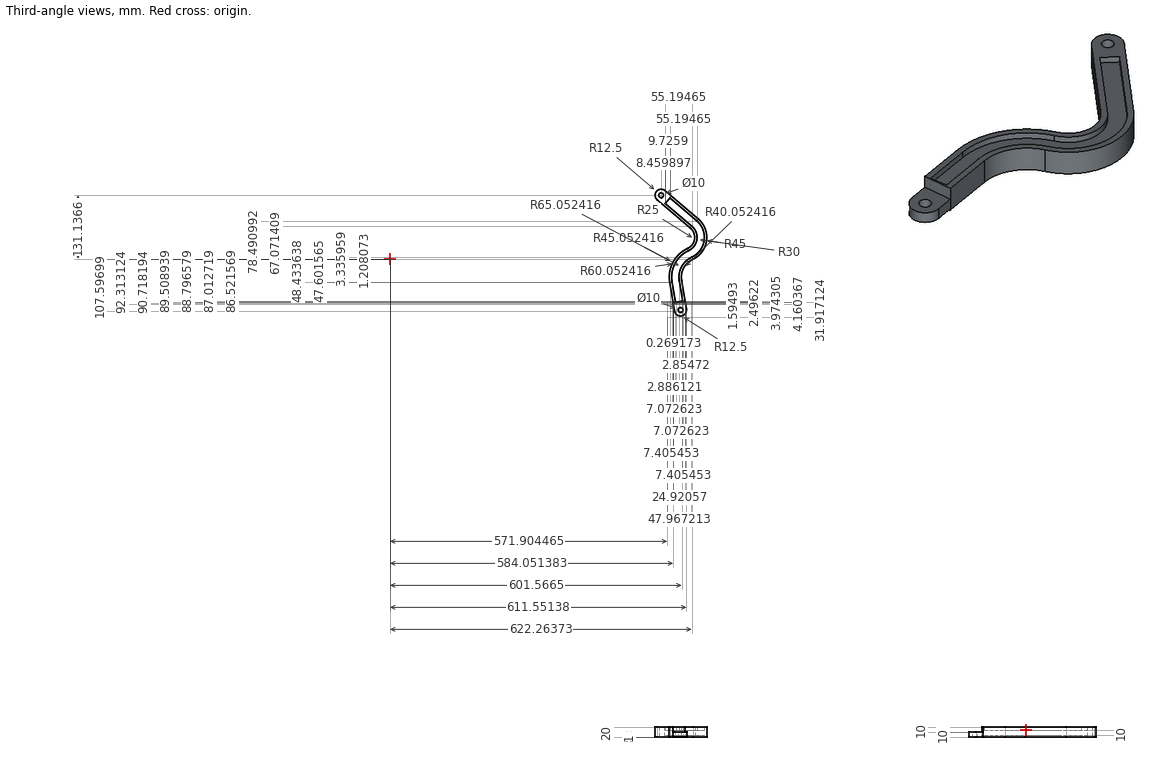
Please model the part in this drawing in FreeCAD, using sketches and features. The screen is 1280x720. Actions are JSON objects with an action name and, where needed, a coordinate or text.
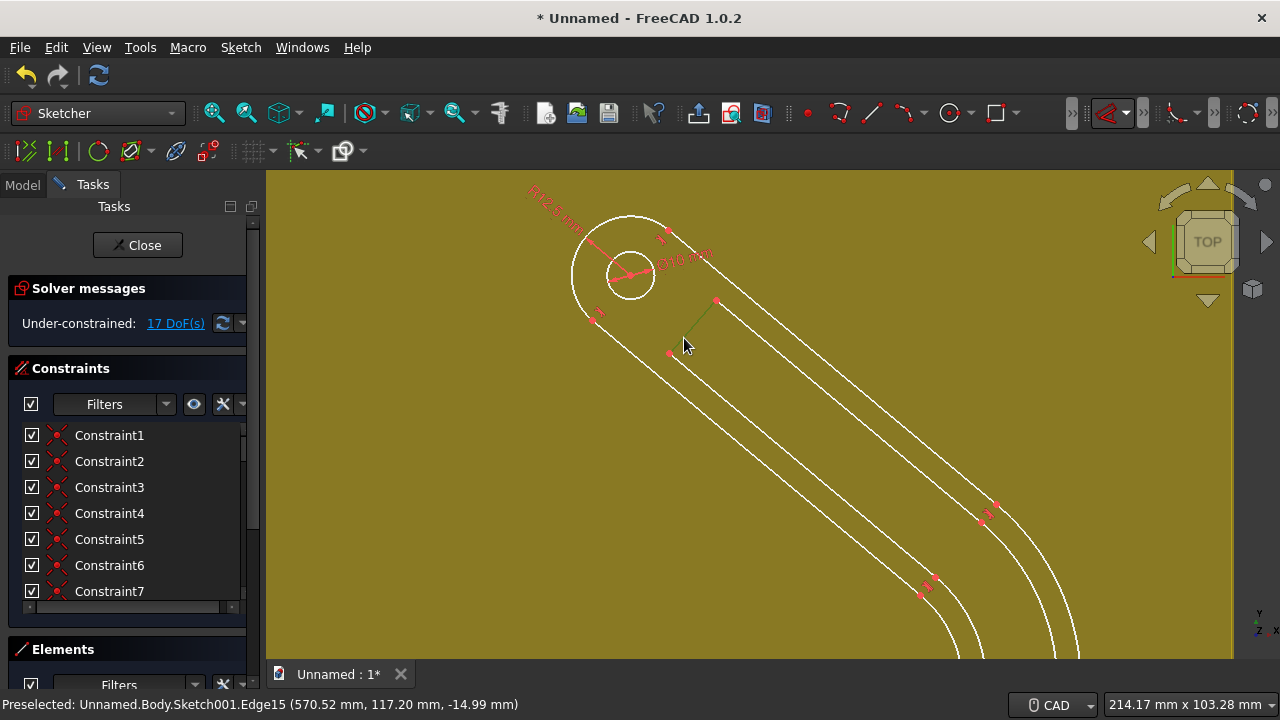
{"action": "key", "text": "l"}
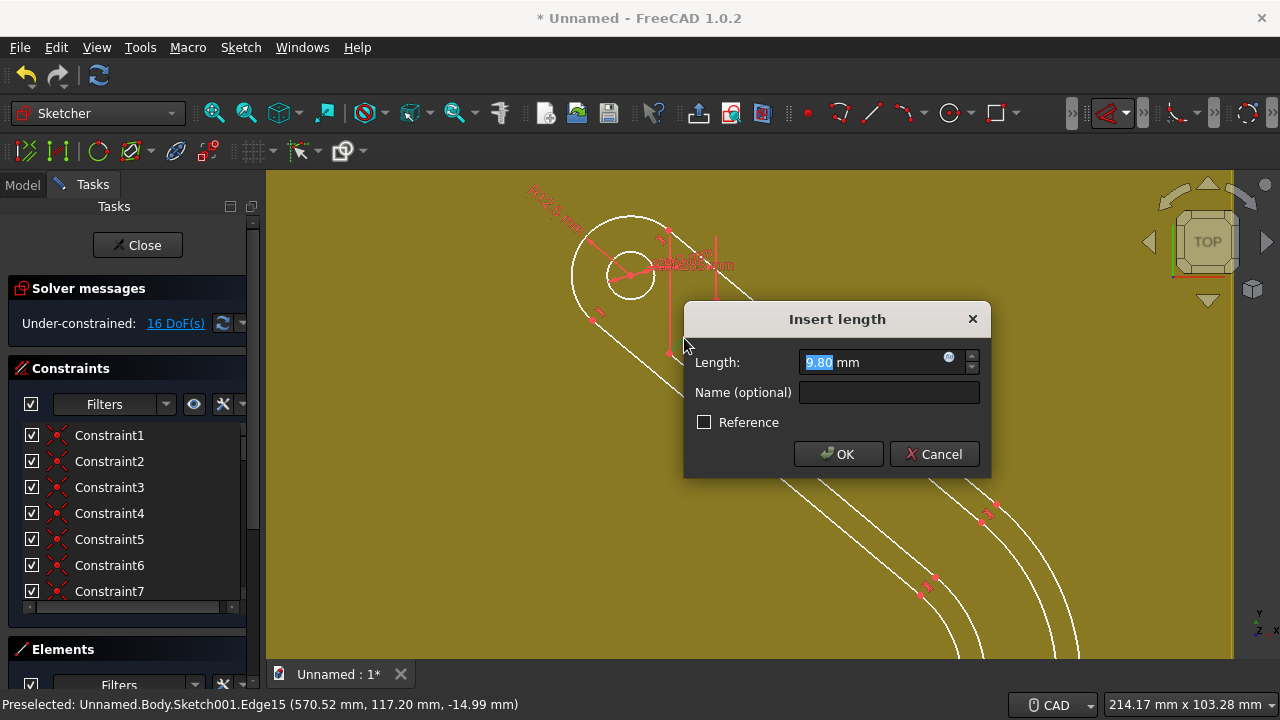
{"action": "type", "text": "9.7259"}
{"action": "key", "text": "Return"}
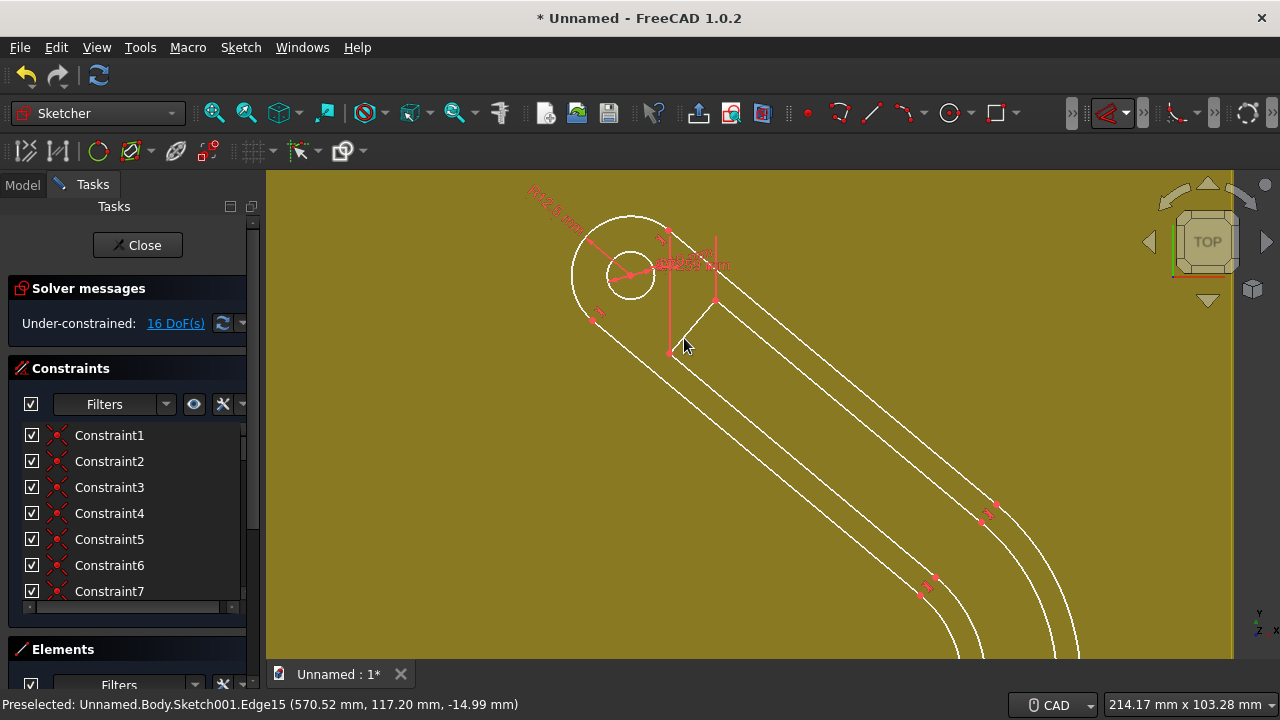
{"action": "scroll", "coordinate": [651, 258], "scroll_direction": "down", "scroll_amount": 6}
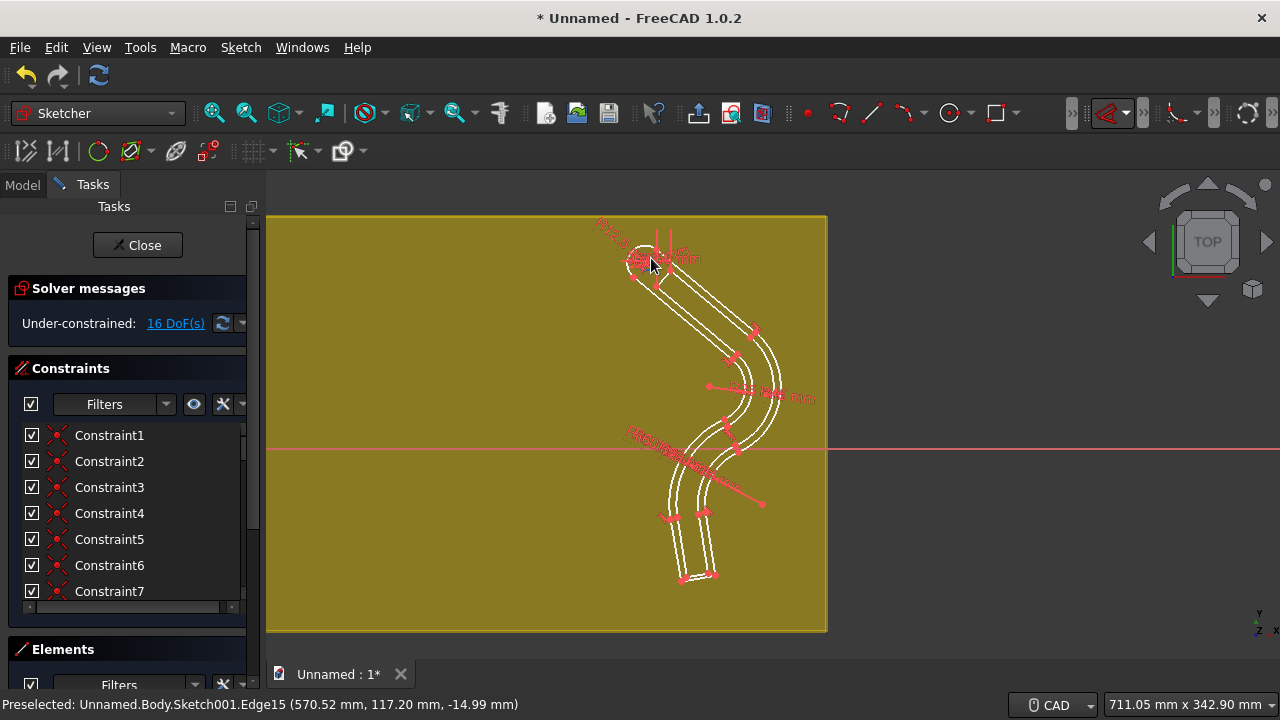
{"action": "scroll", "coordinate": [702, 575], "scroll_direction": "up", "scroll_amount": 13}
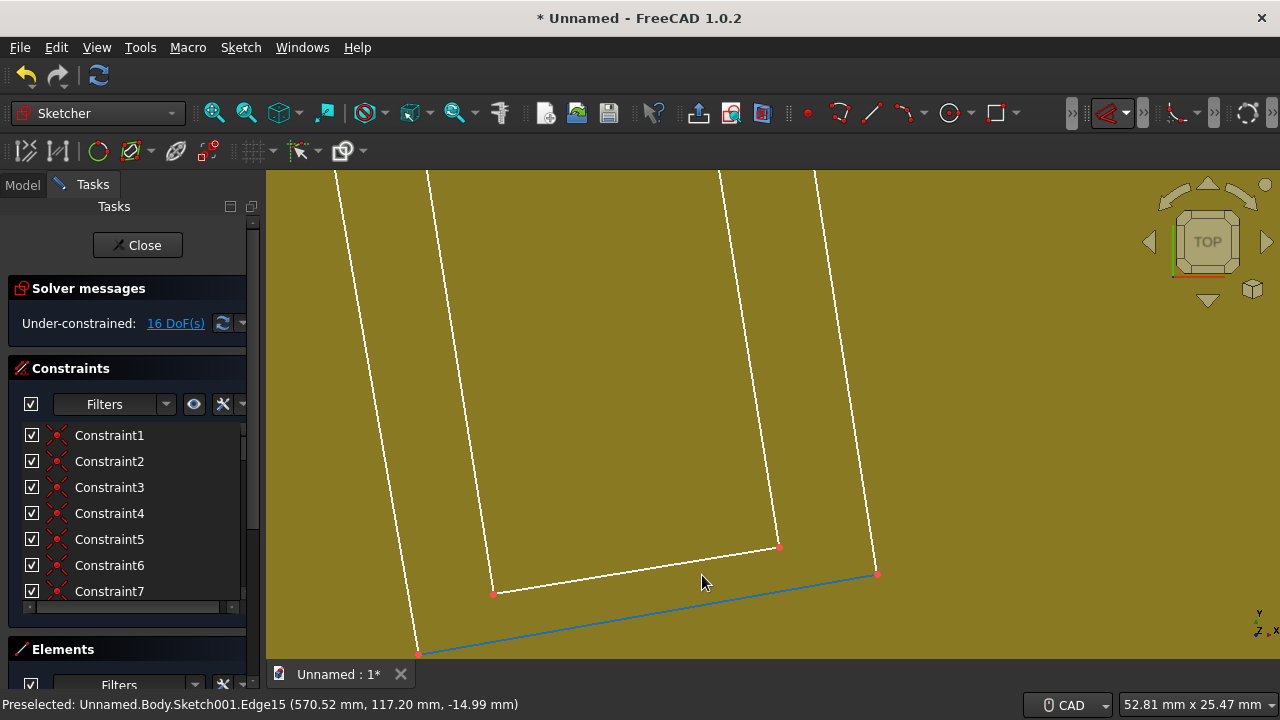
{"action": "left_click", "coordinate": [694, 561]}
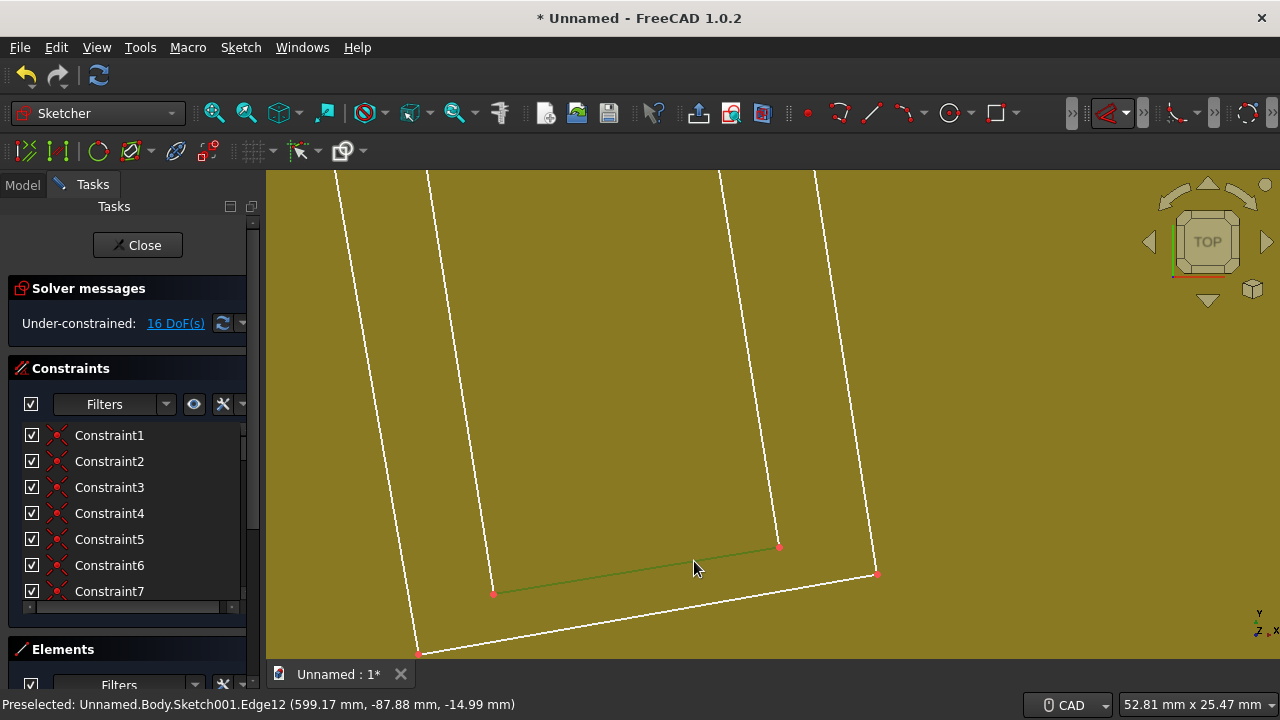
{"action": "left_click", "coordinate": [1128, 114]}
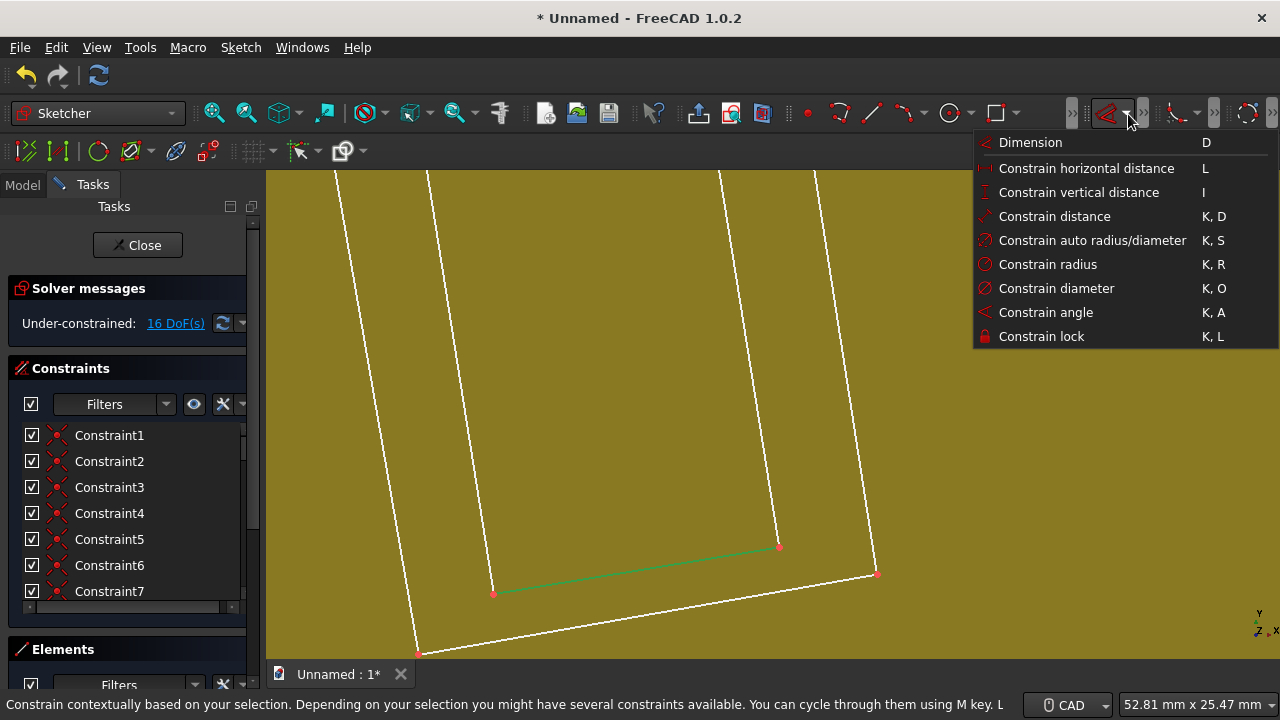
{"action": "left_click", "coordinate": [1126, 192]}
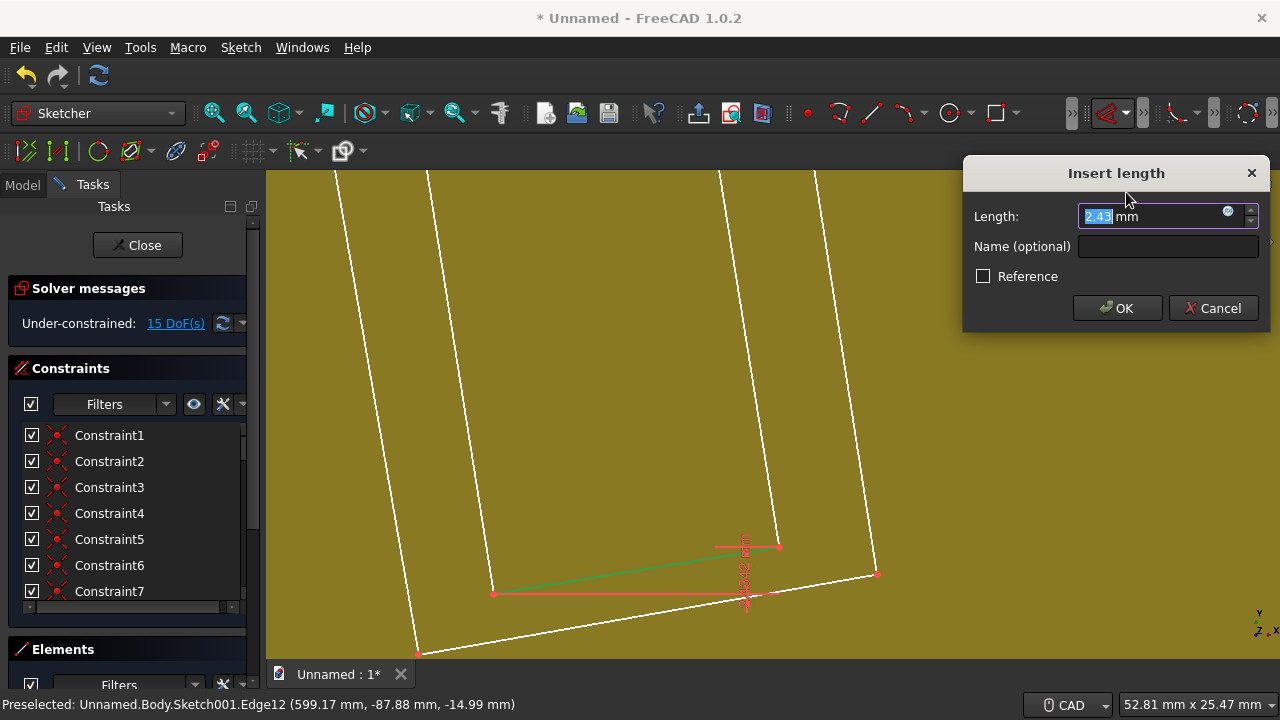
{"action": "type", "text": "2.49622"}
{"action": "key", "text": "Return"}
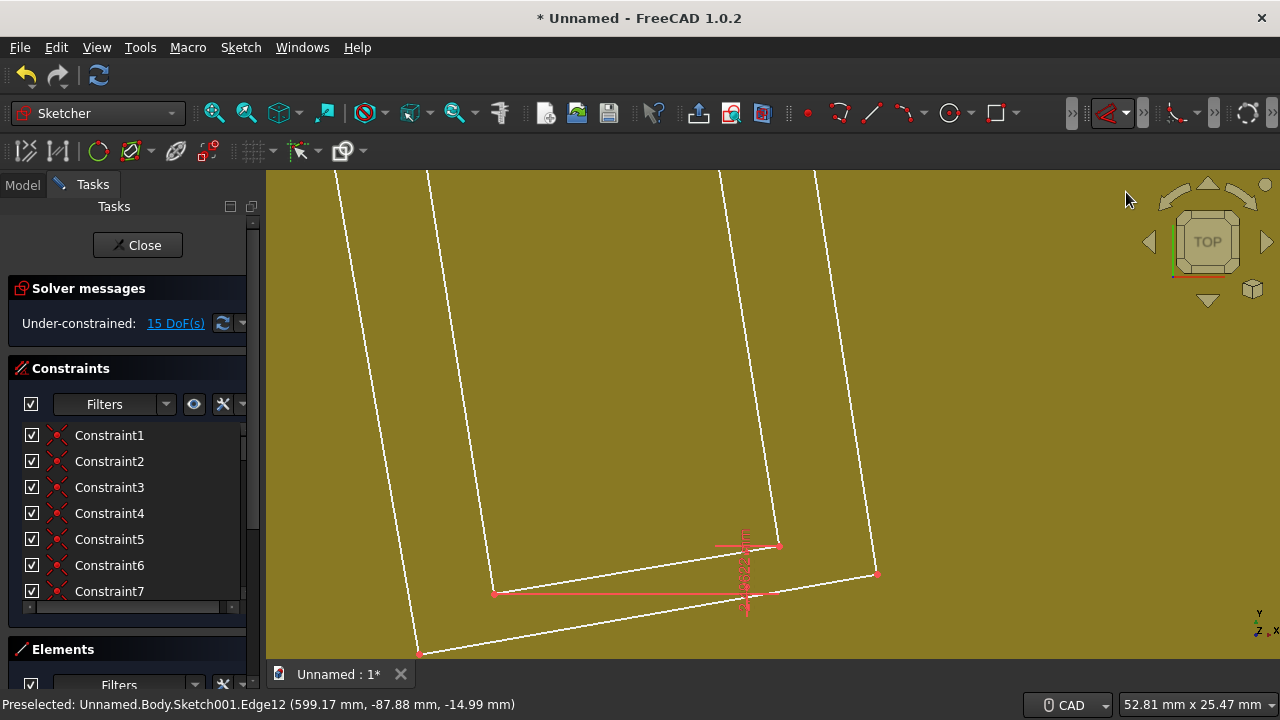
{"action": "scroll", "coordinate": [702, 575], "scroll_direction": "down", "scroll_amount": 13}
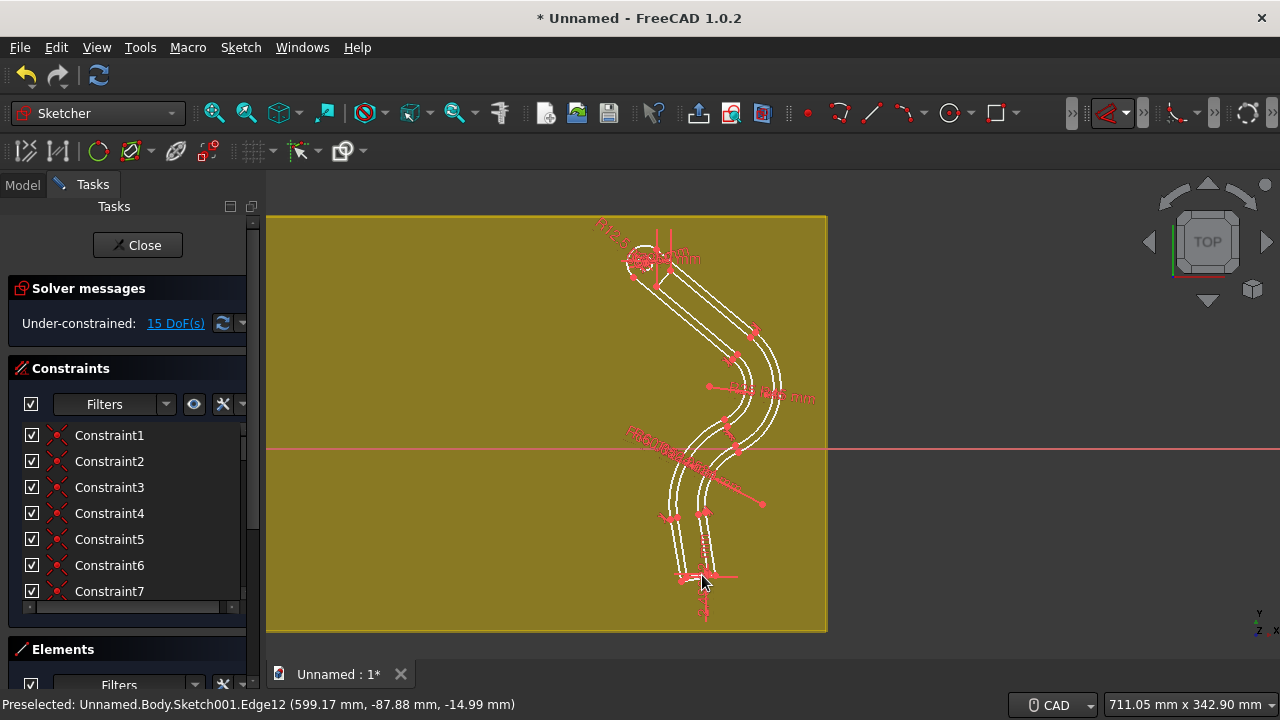
{"action": "left_click", "coordinate": [645, 263]}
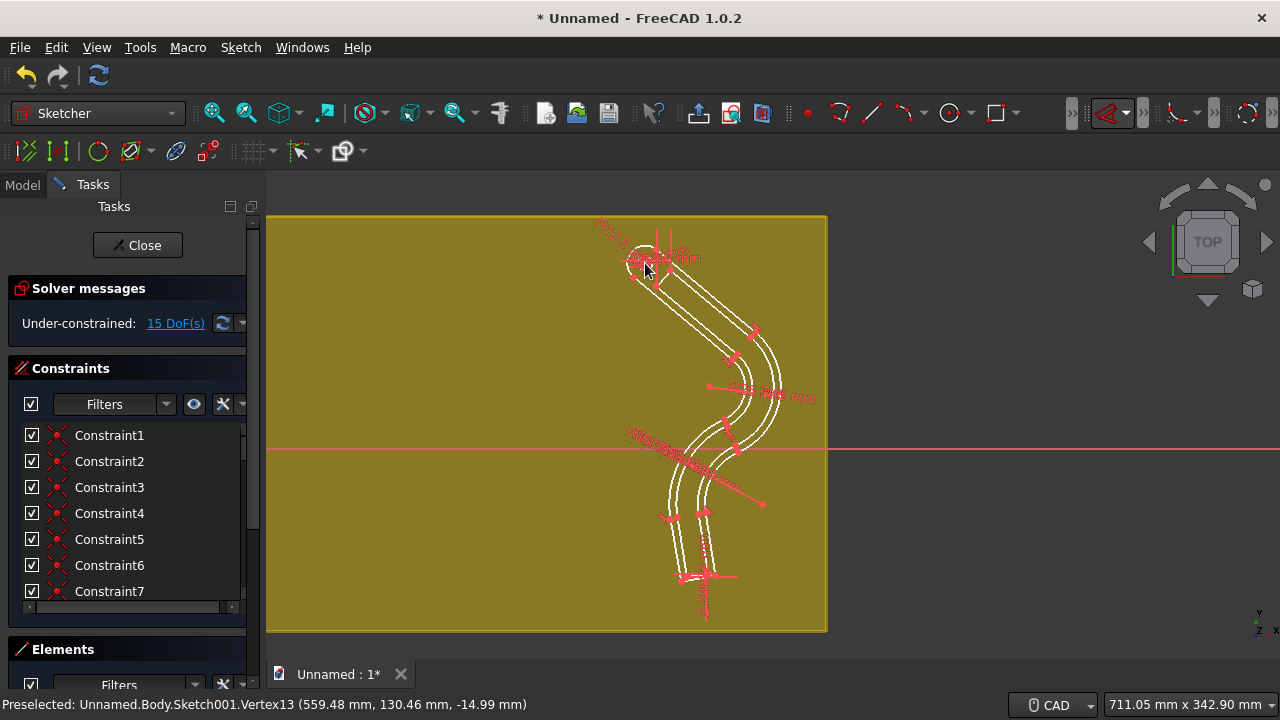
{"action": "key", "text": "i"}